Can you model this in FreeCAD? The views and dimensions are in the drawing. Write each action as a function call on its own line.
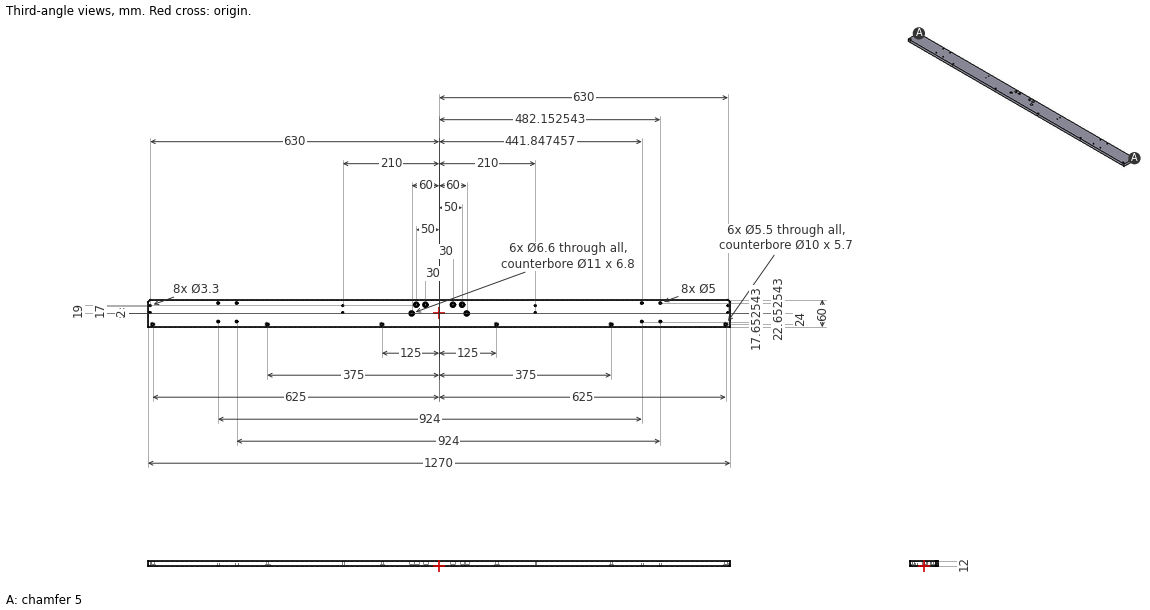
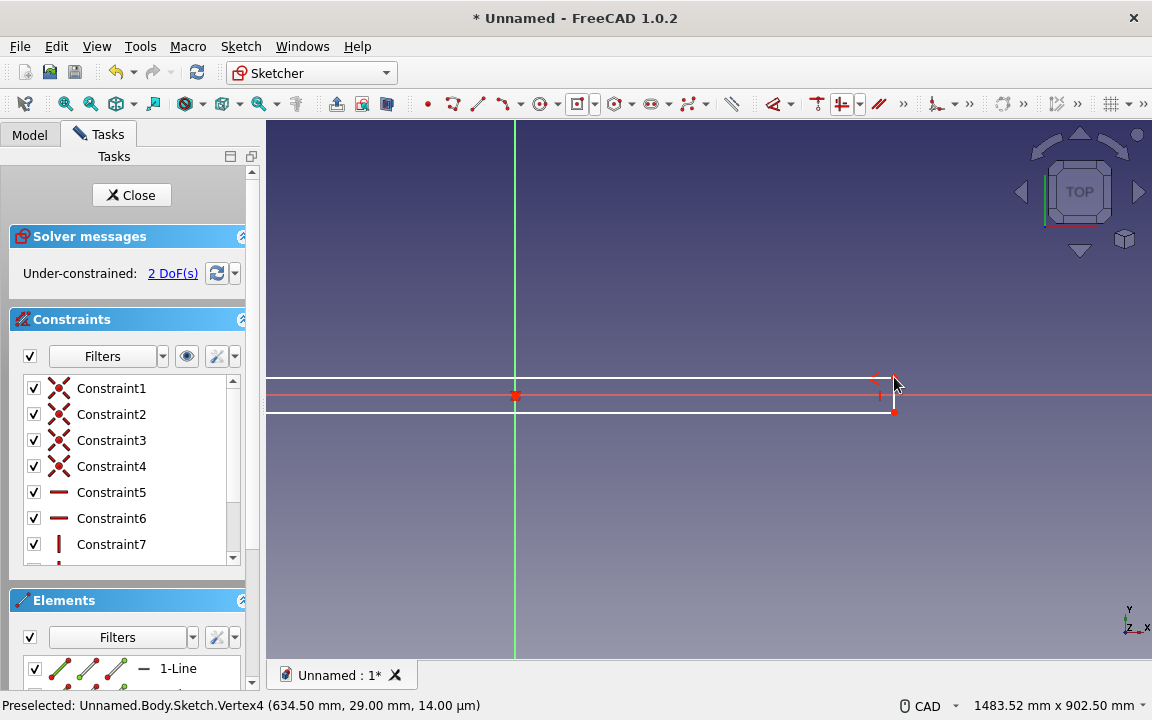
click(894, 399)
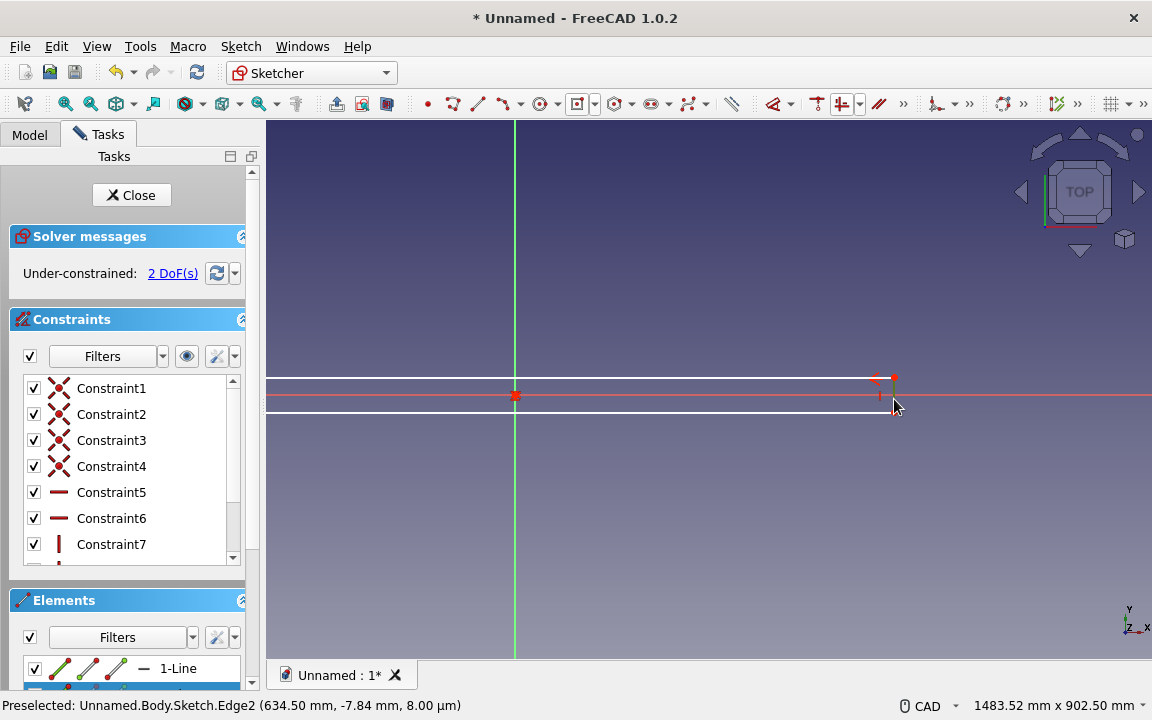
key(i)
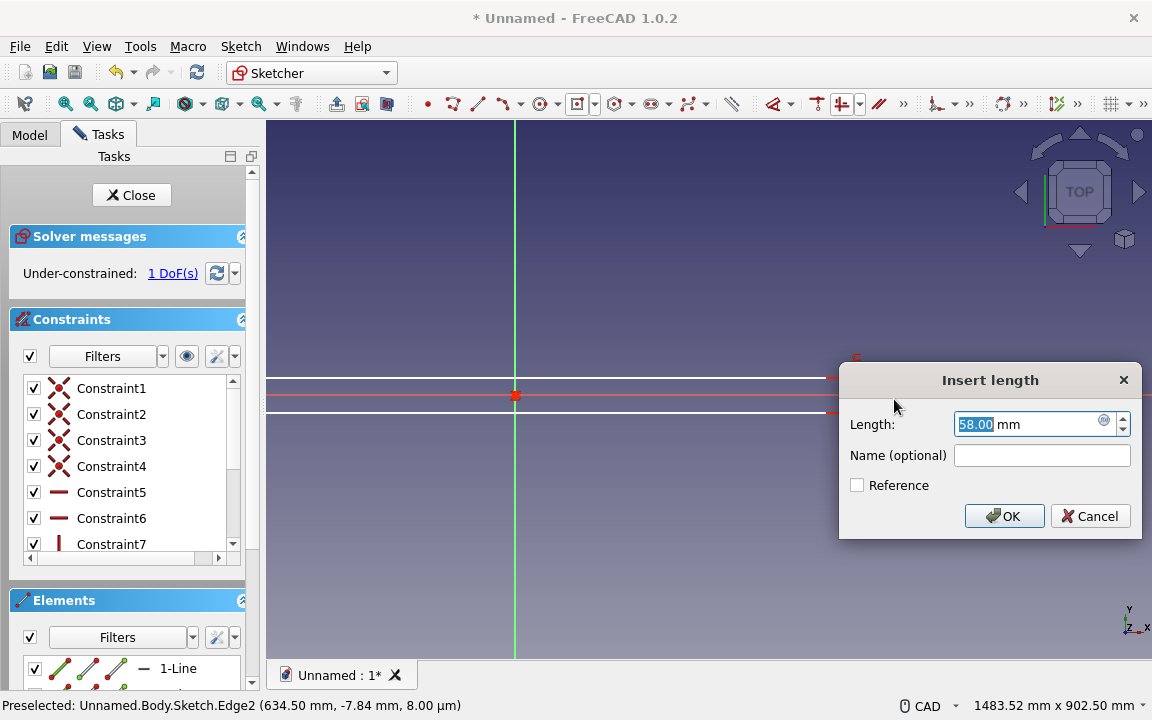
text(60)
key(Return)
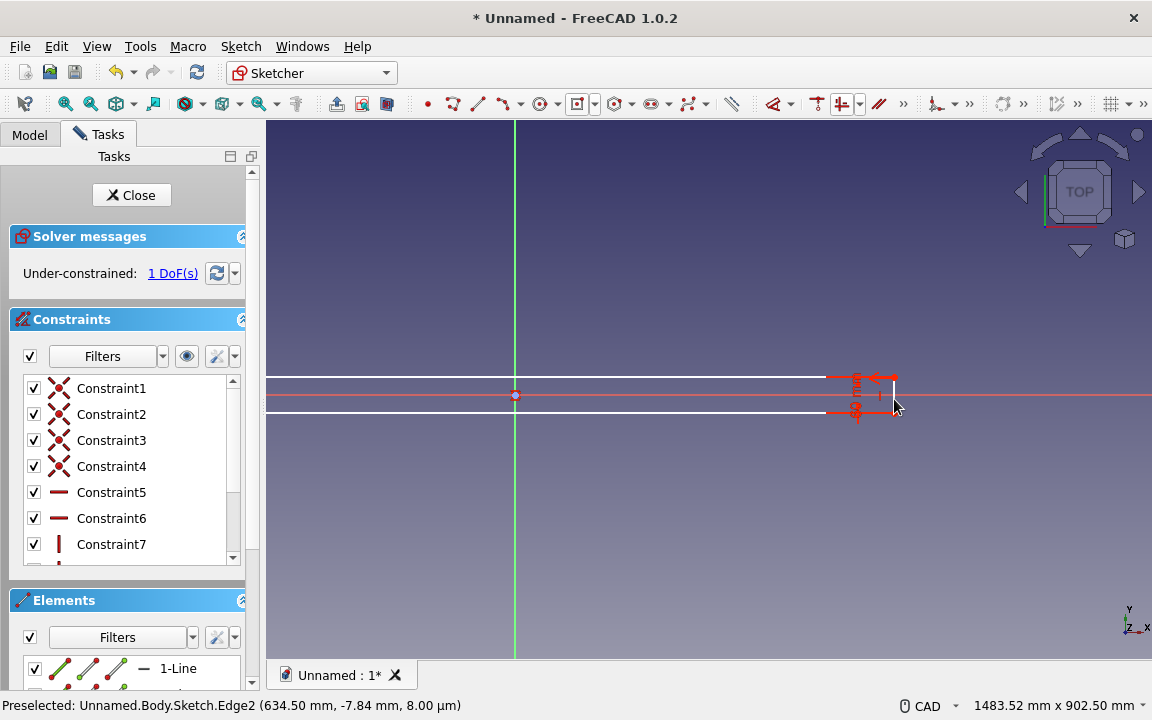
click(363, 413)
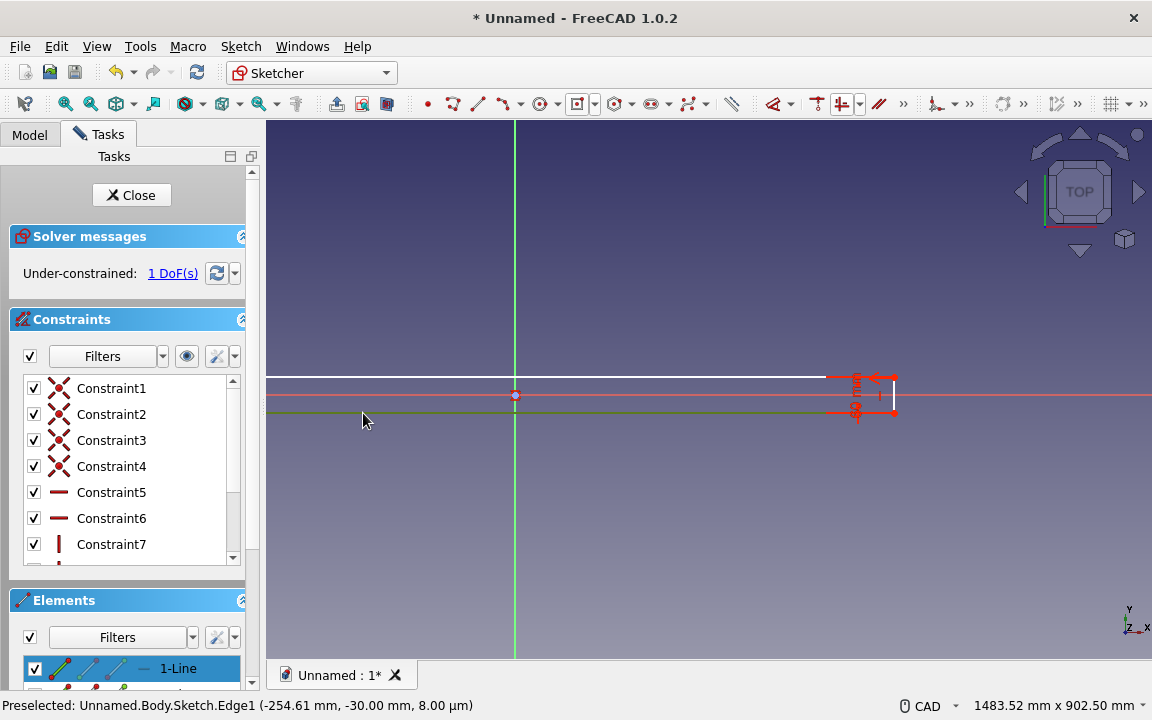
click(790, 104)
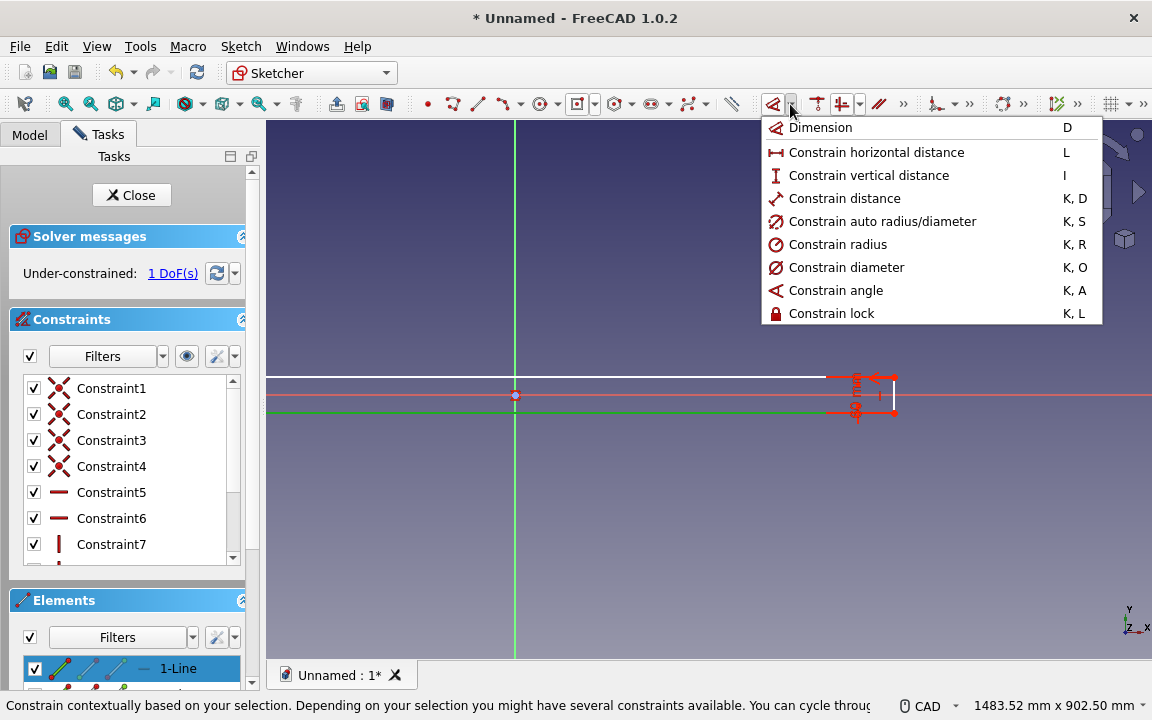
click(932, 152)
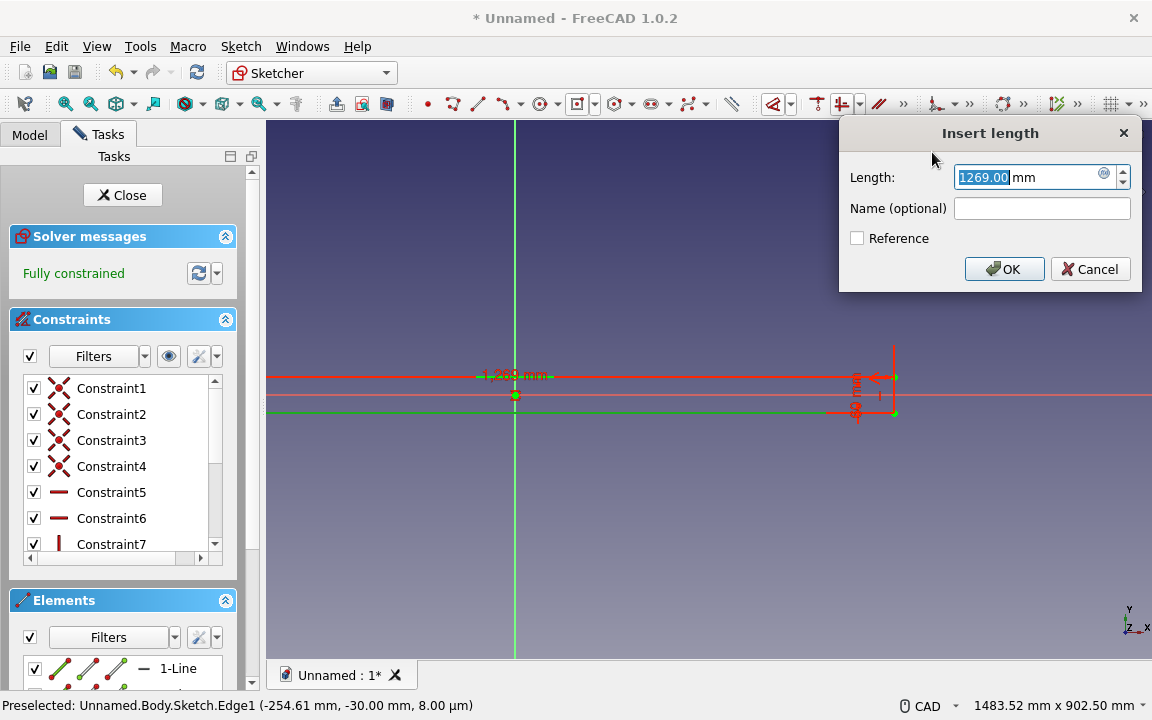
text(1270)
key(Return)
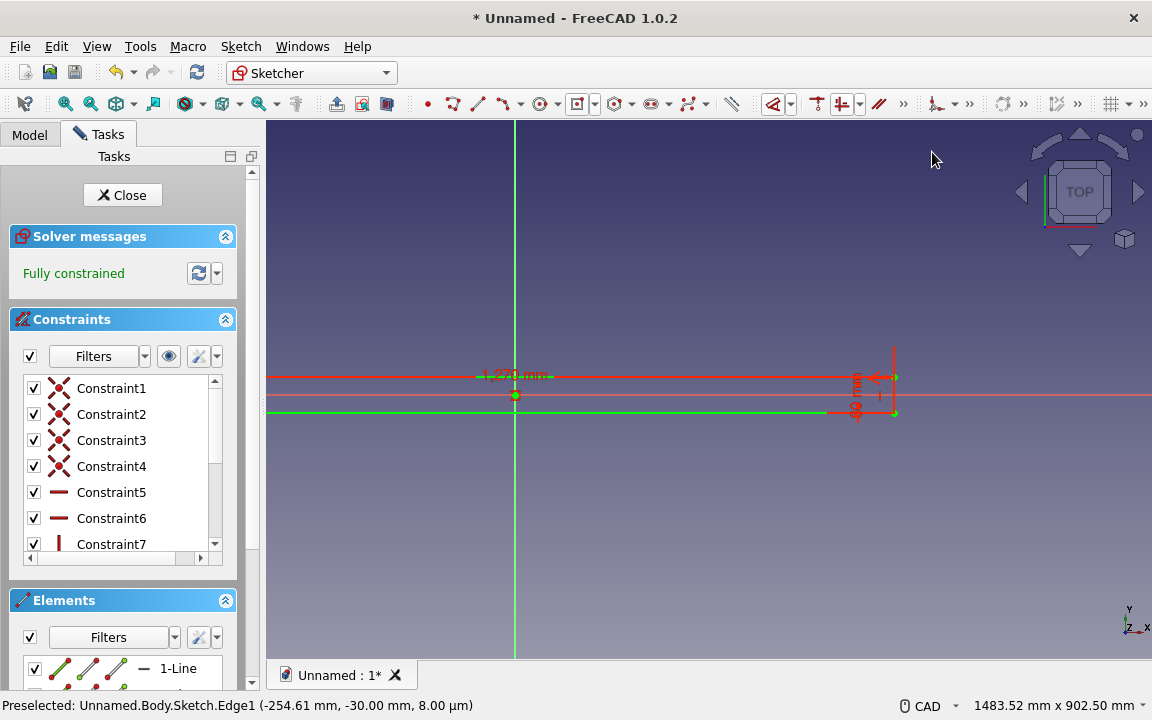
click(123, 195)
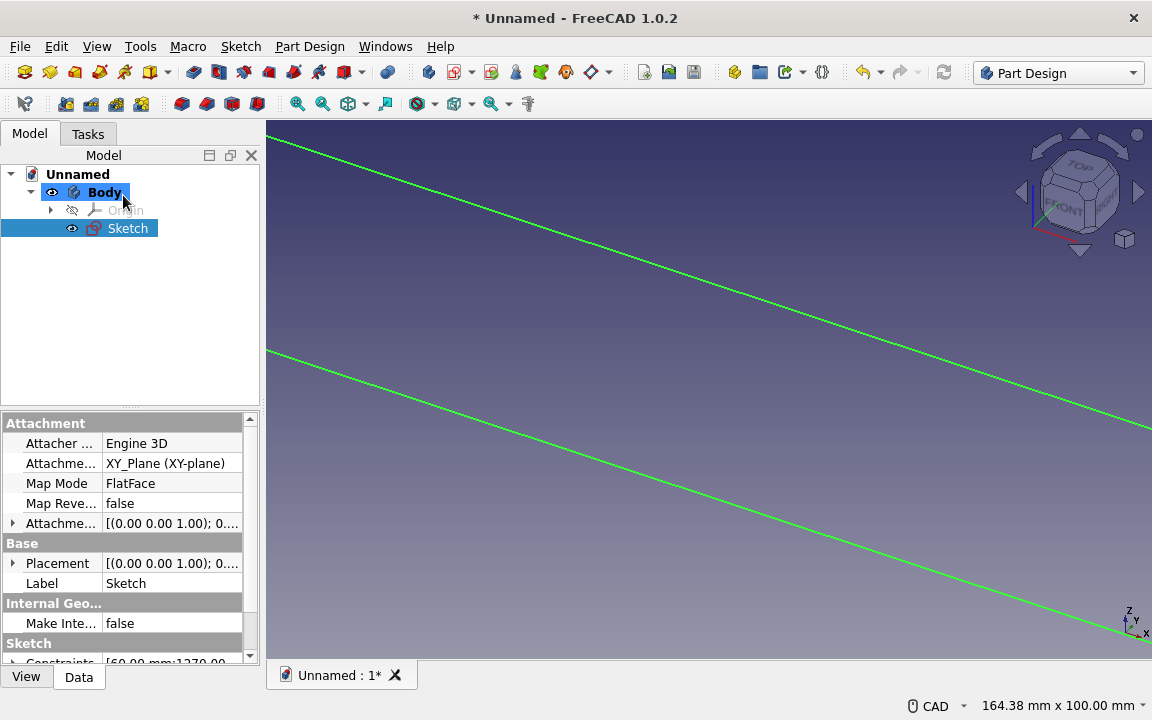
click(25, 72)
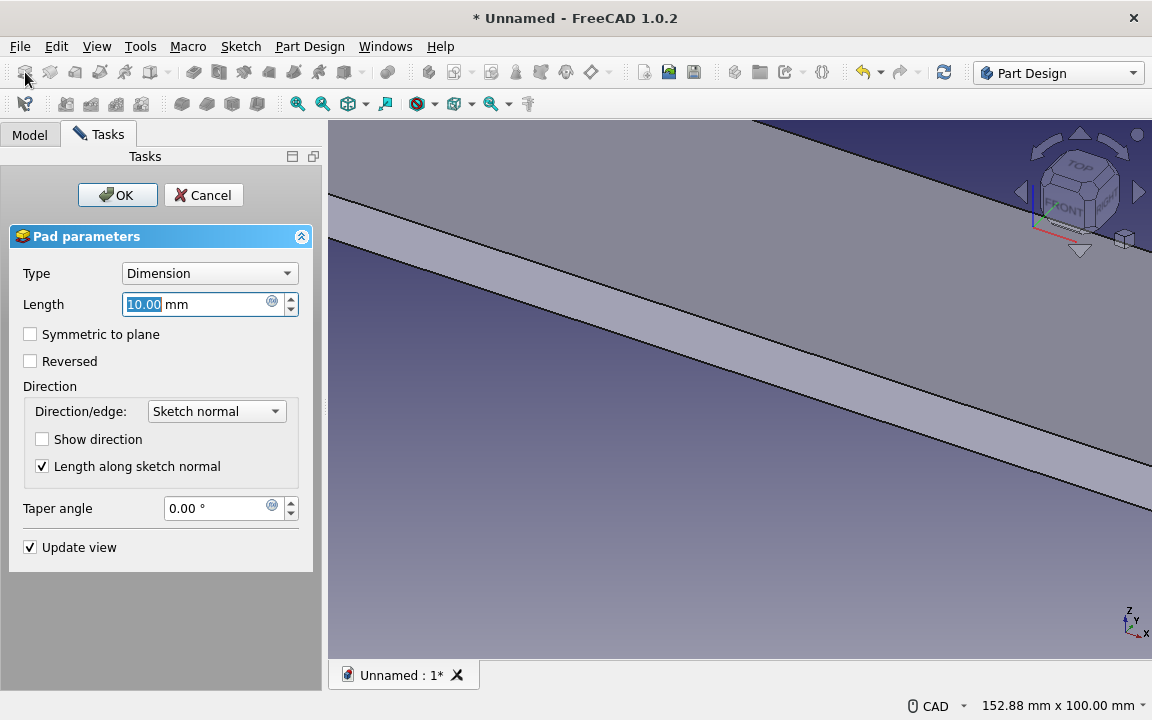
text(12)
key(Tab)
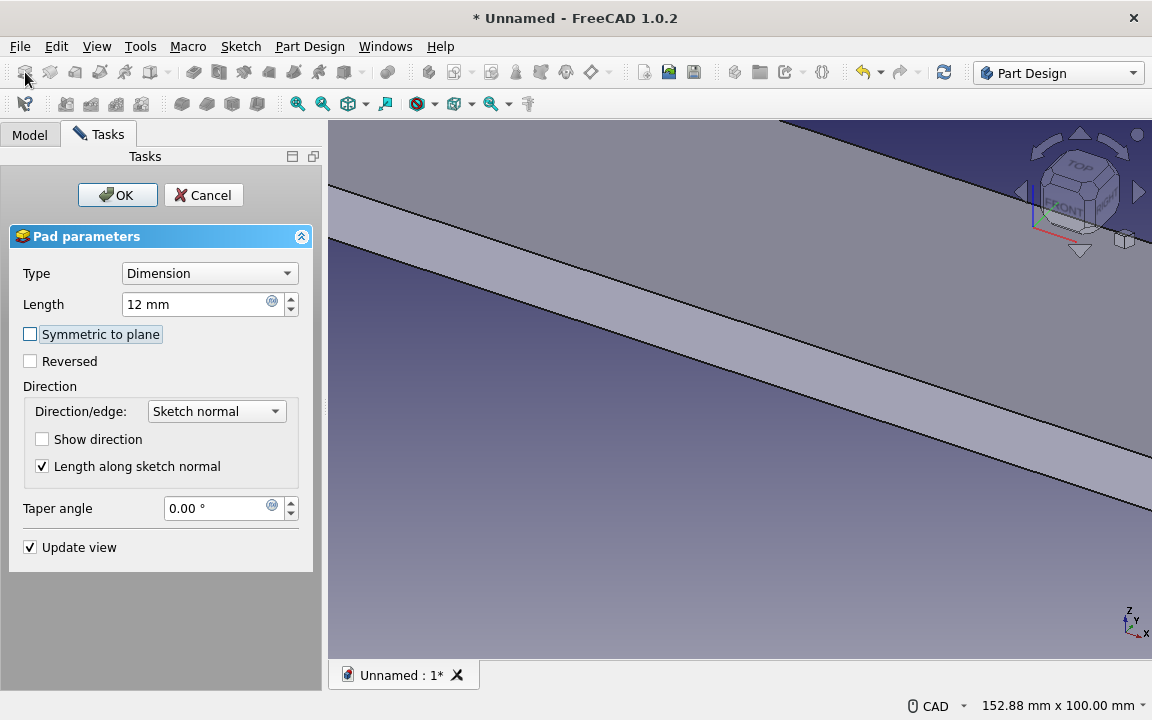
click(118, 195)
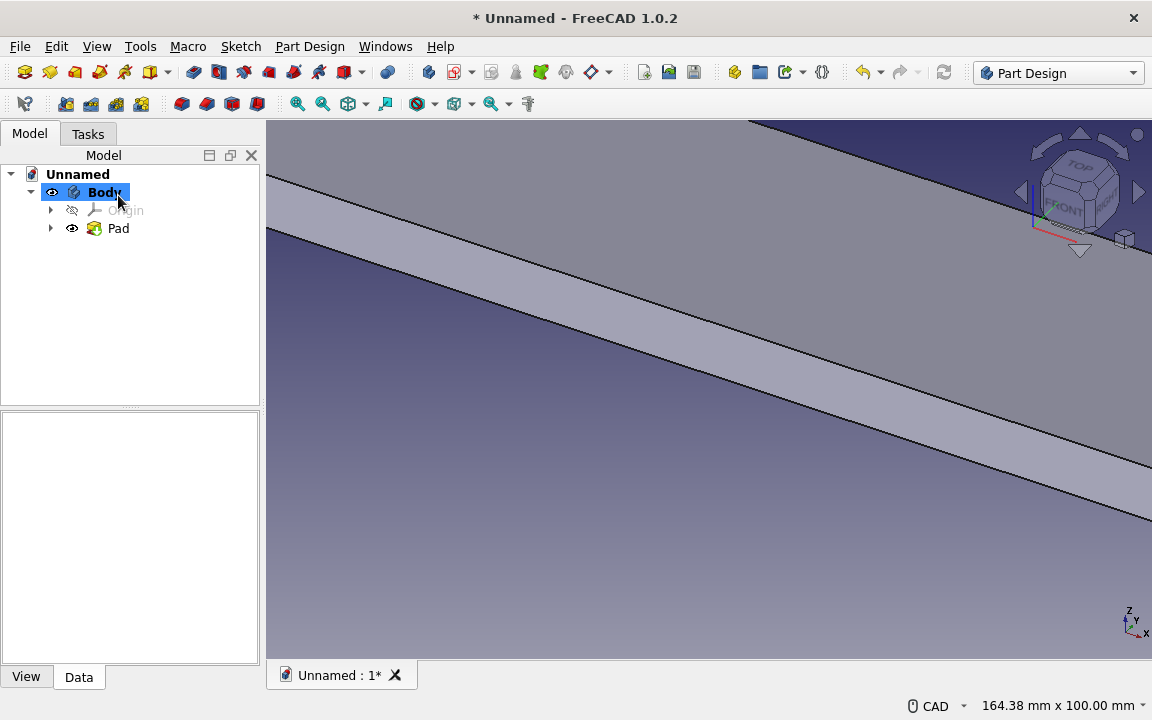
click(298, 104)